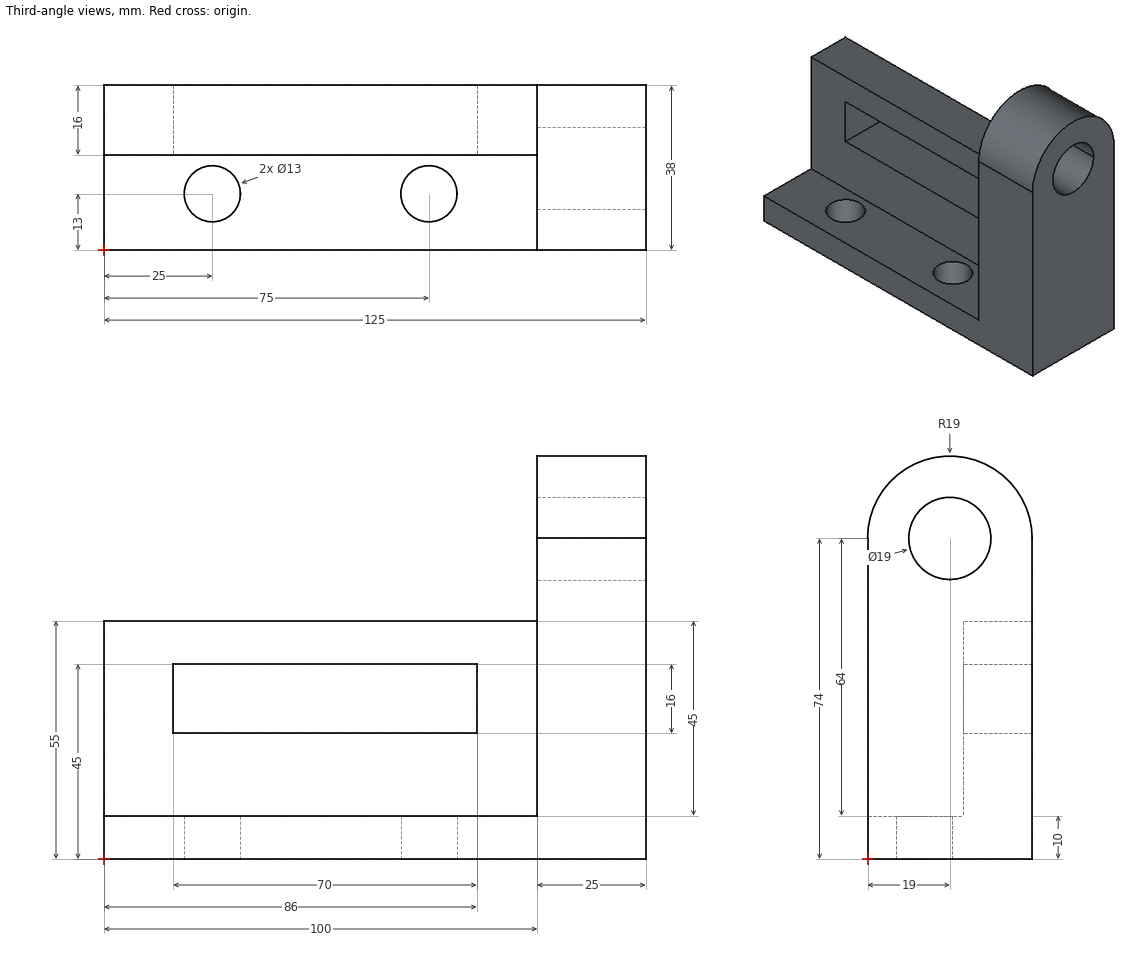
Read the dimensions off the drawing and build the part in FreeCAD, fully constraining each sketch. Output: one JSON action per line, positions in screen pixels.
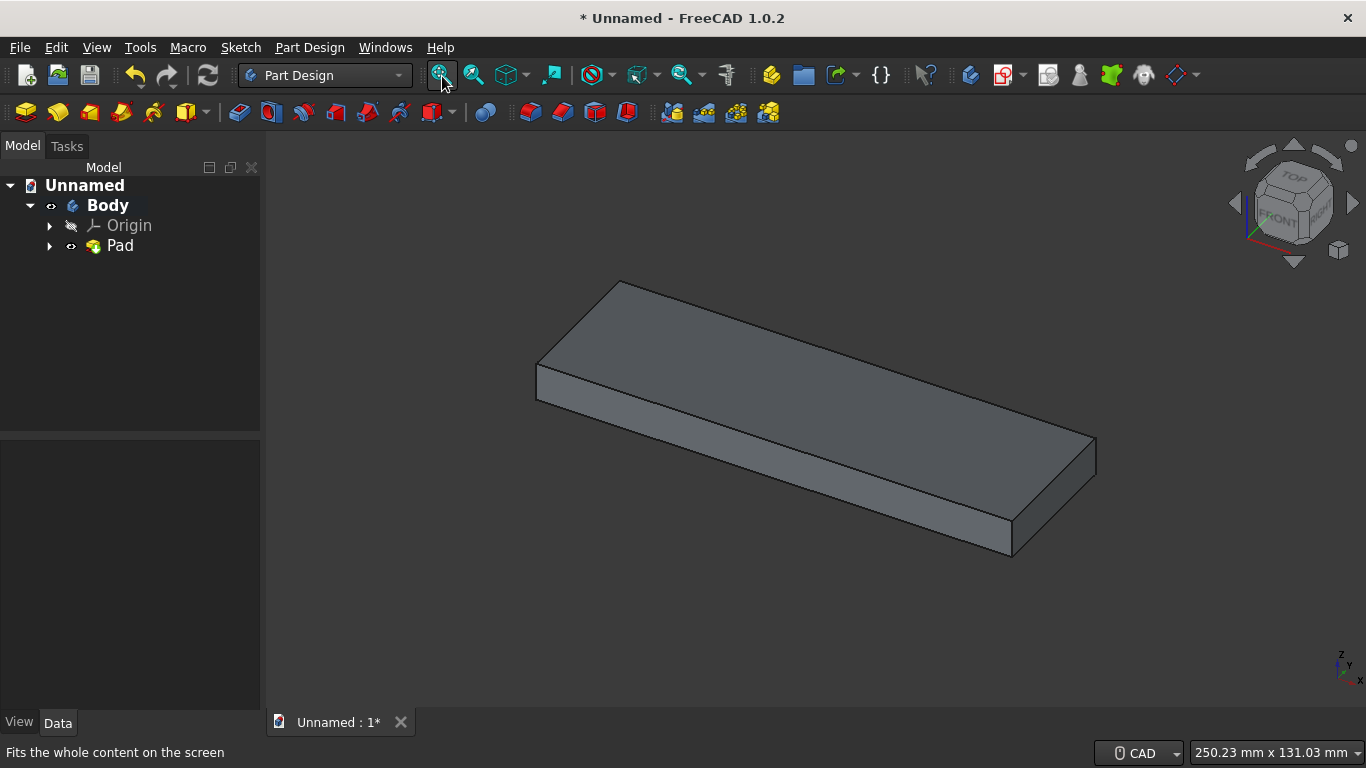
{"action": "left_click", "coordinate": [1078, 473]}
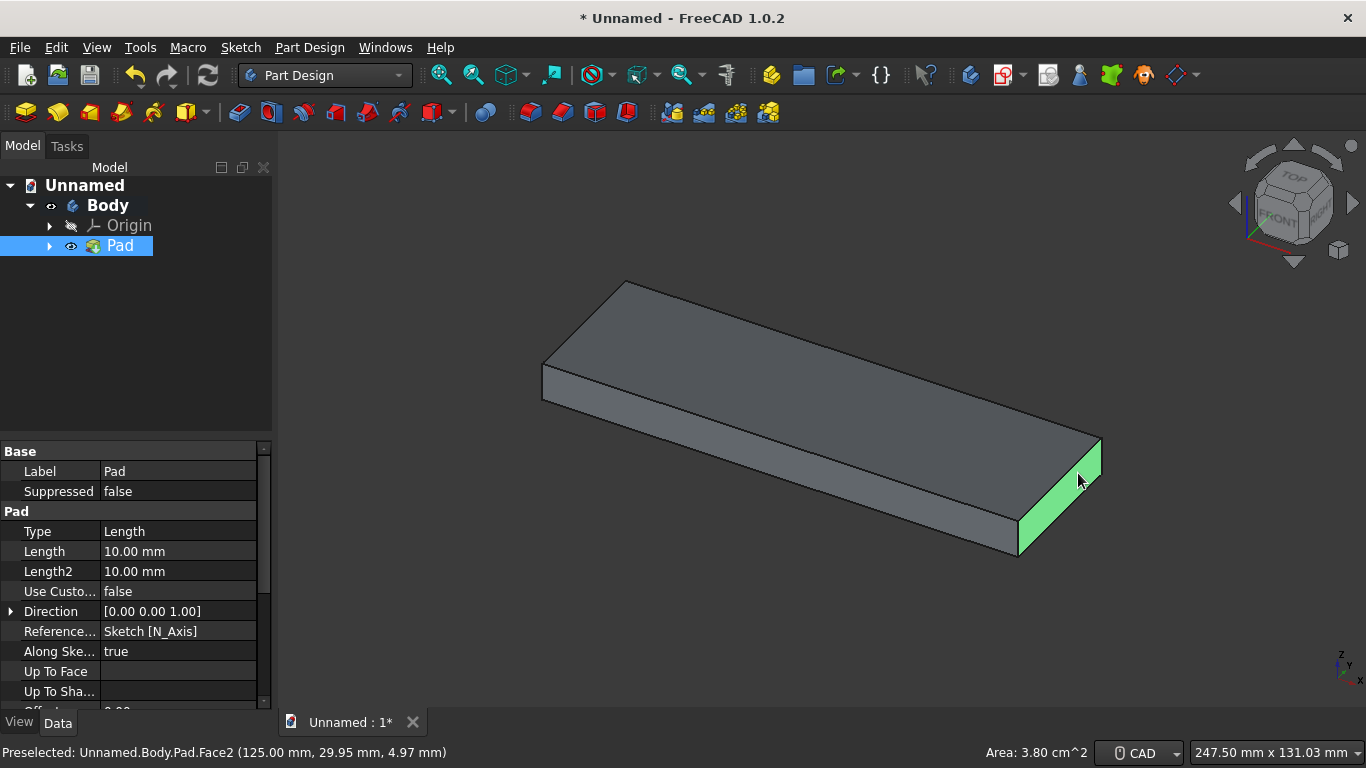
{"action": "left_click", "coordinate": [1004, 76]}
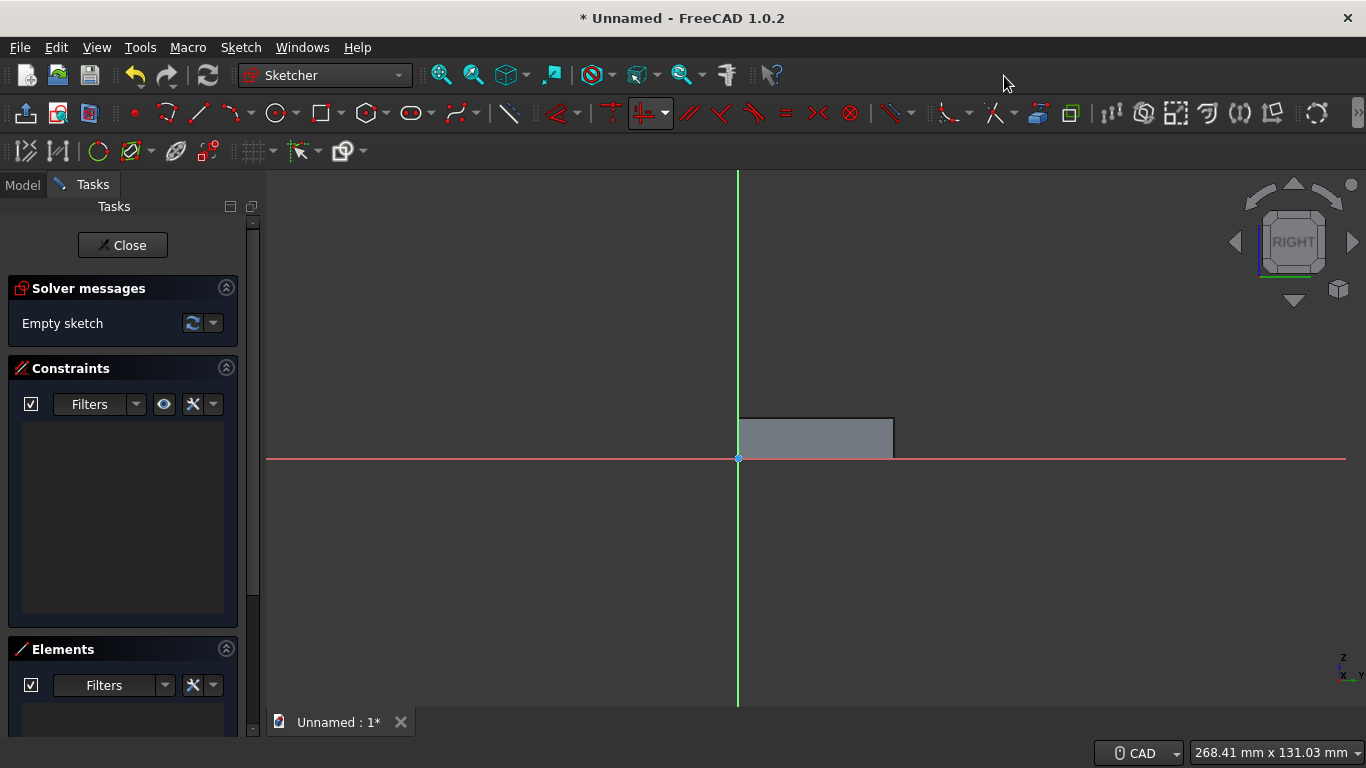
{"action": "scroll", "coordinate": [608, 679], "scroll_direction": "down", "scroll_amount": 2}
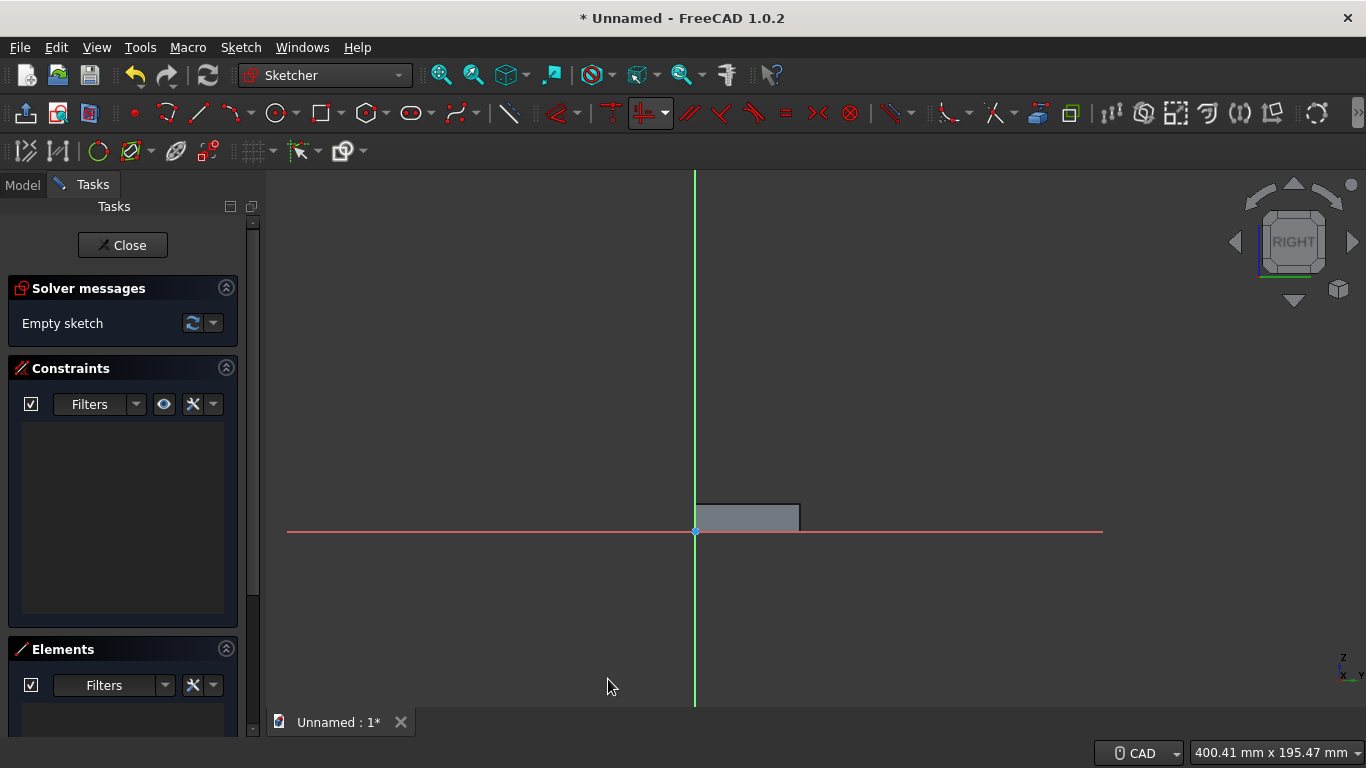
{"action": "left_click", "coordinate": [168, 114]}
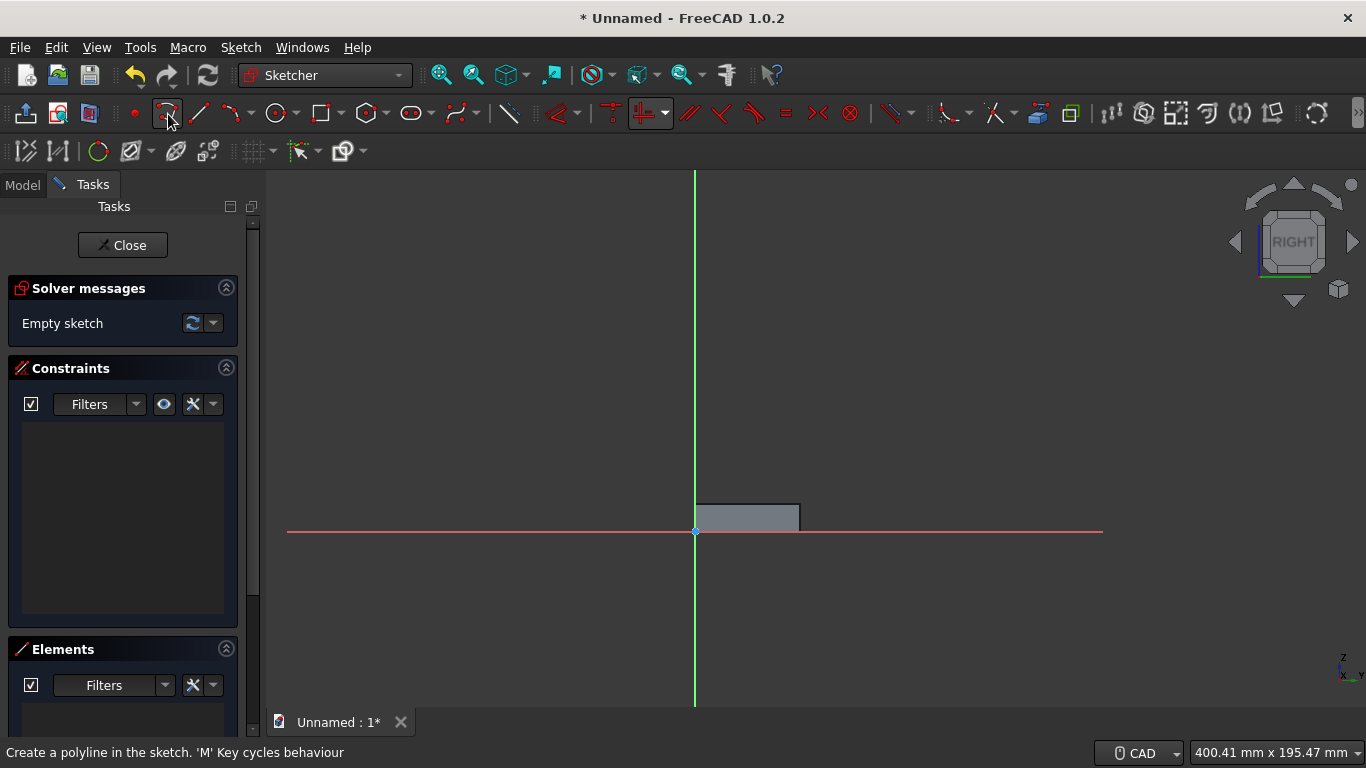
{"action": "left_click", "coordinate": [695, 329]}
{"action": "left_click", "coordinate": [704, 504]}
{"action": "left_click", "coordinate": [800, 504]}
{"action": "left_click", "coordinate": [800, 329]}
{"action": "right_click", "coordinate": [800, 329]}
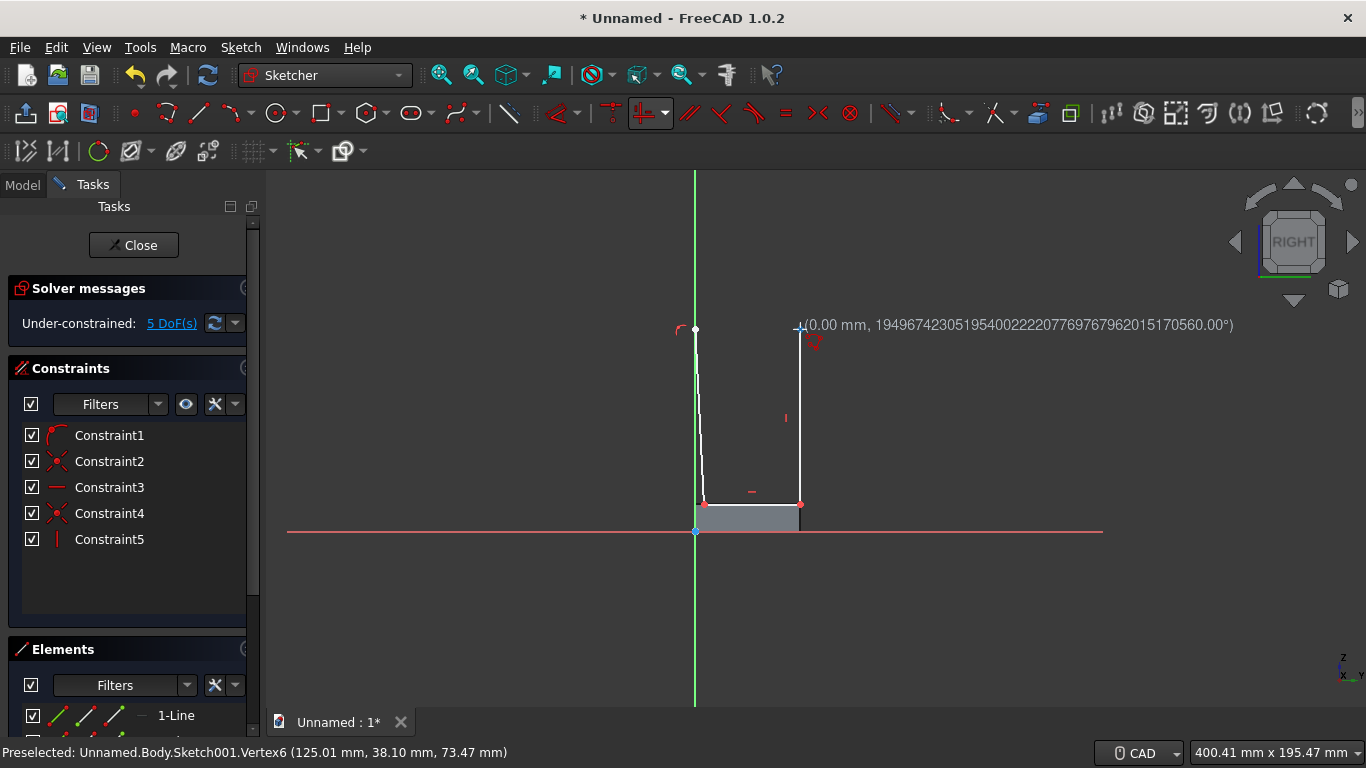
{"action": "left_click", "coordinate": [232, 114]}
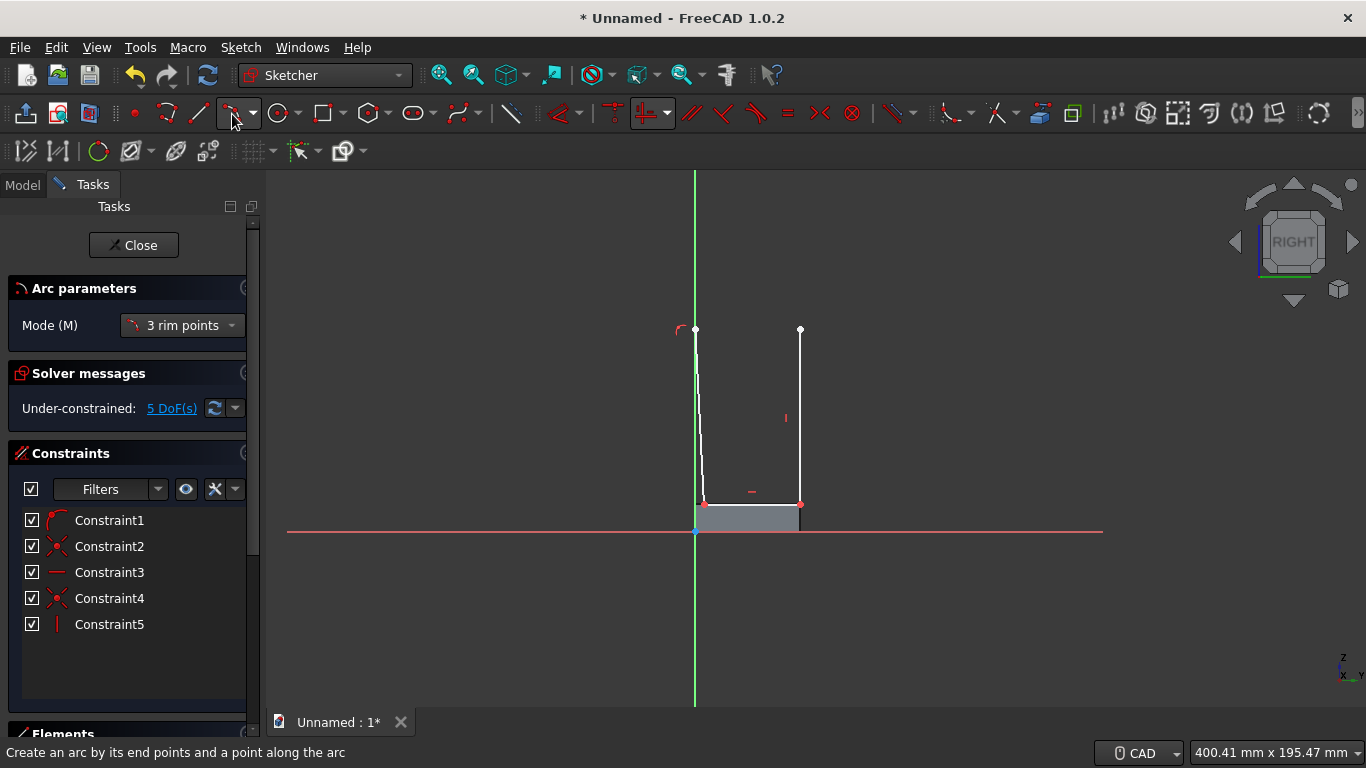
{"action": "left_click", "coordinate": [800, 330]}
{"action": "left_click", "coordinate": [695, 330]}
{"action": "left_click", "coordinate": [748, 276]}
{"action": "key", "text": "Escape"}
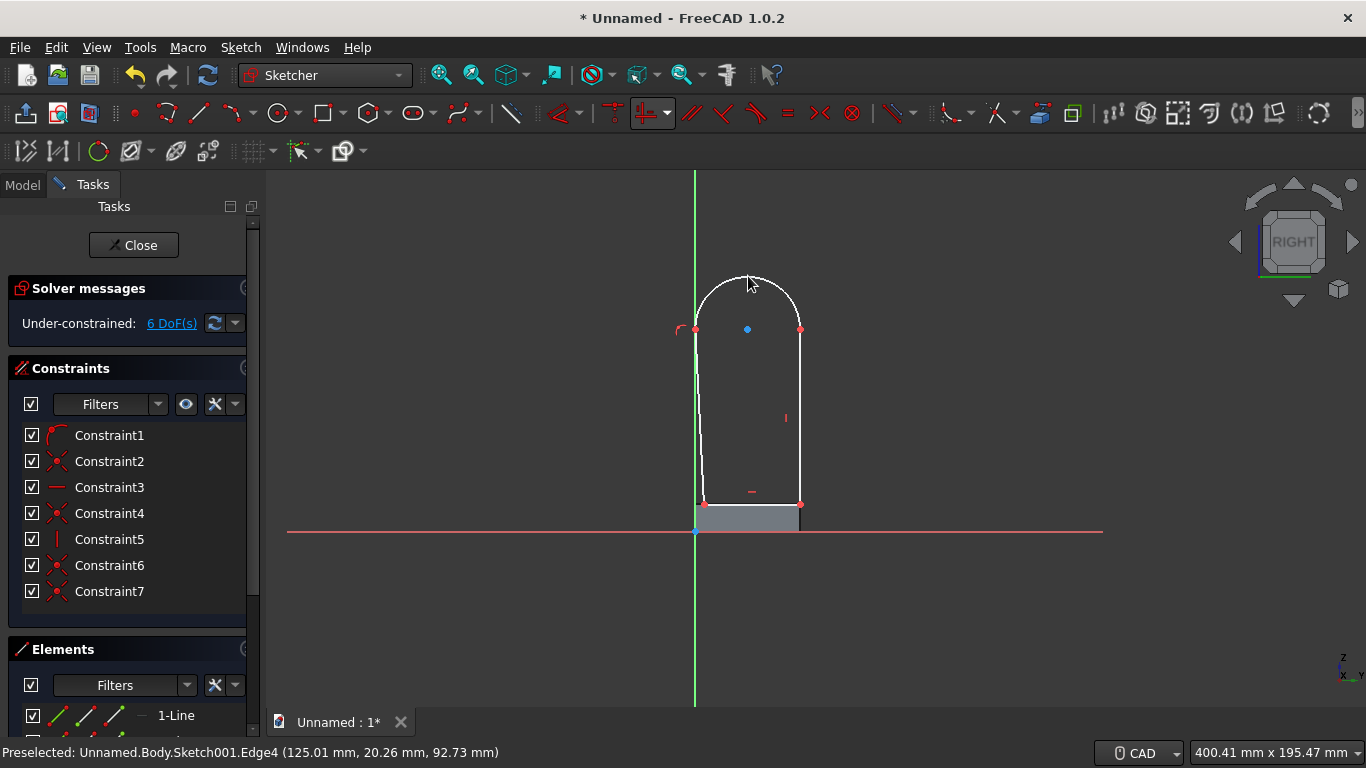
{"action": "left_click", "coordinate": [698, 383]}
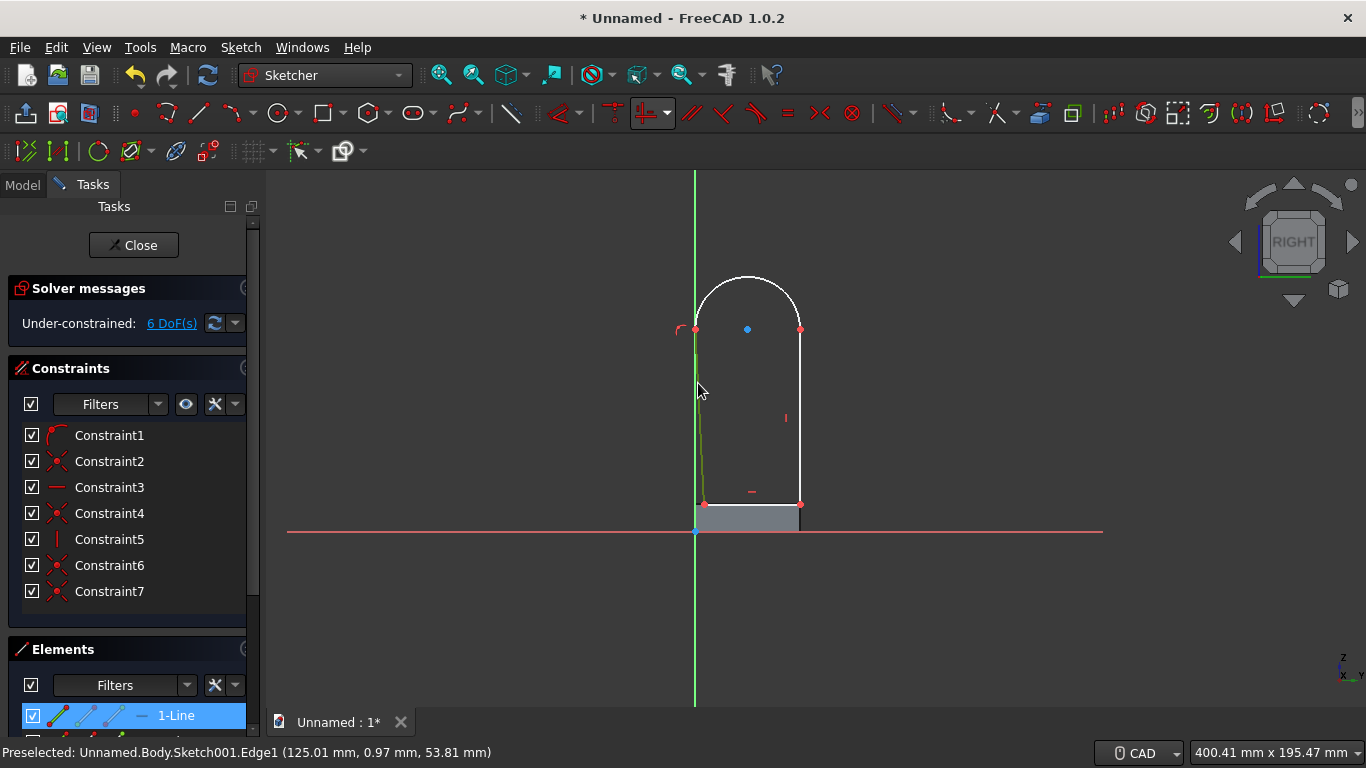
{"action": "left_click", "coordinate": [779, 287]}